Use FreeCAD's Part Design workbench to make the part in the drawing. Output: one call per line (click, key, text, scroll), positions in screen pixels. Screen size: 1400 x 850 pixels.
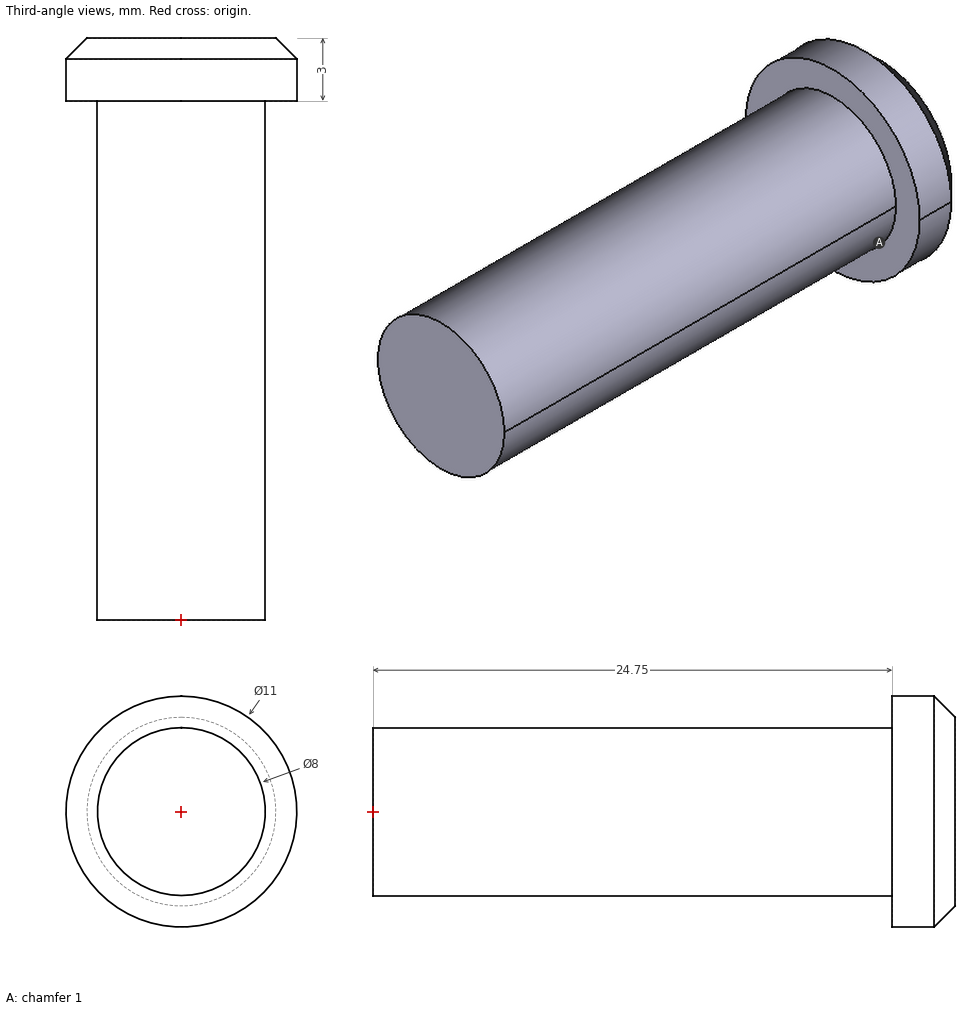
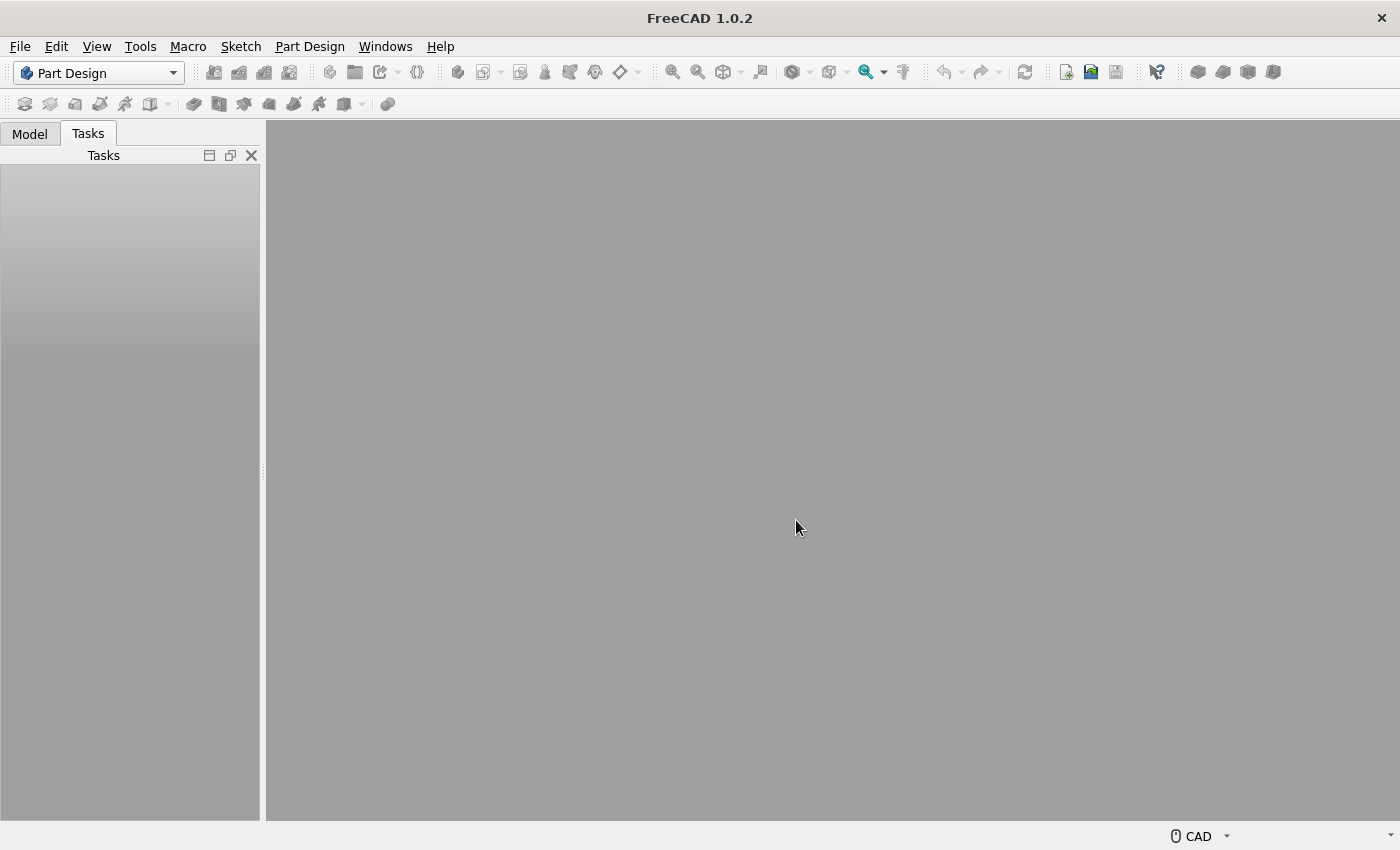
click(1066, 72)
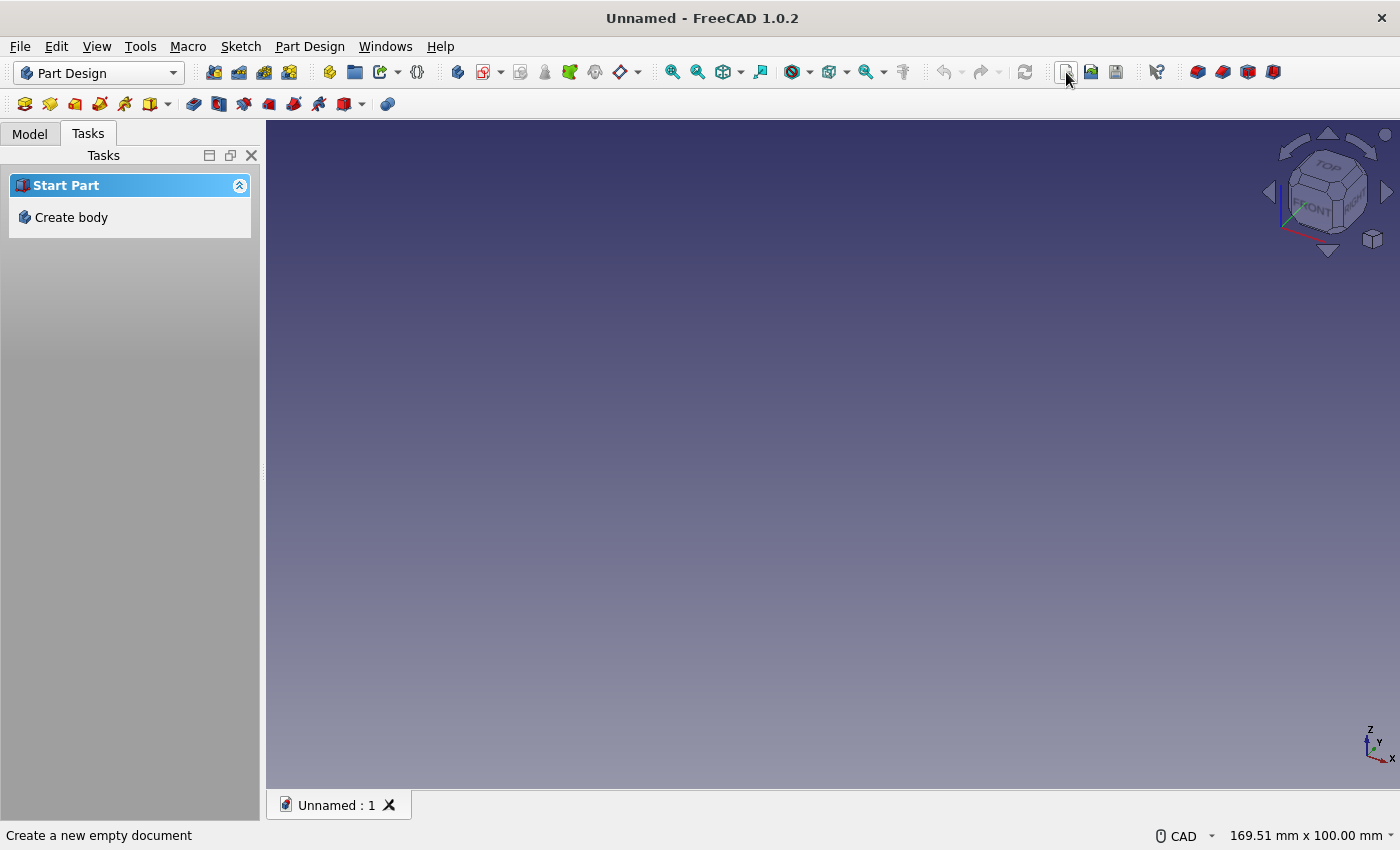
click(482, 72)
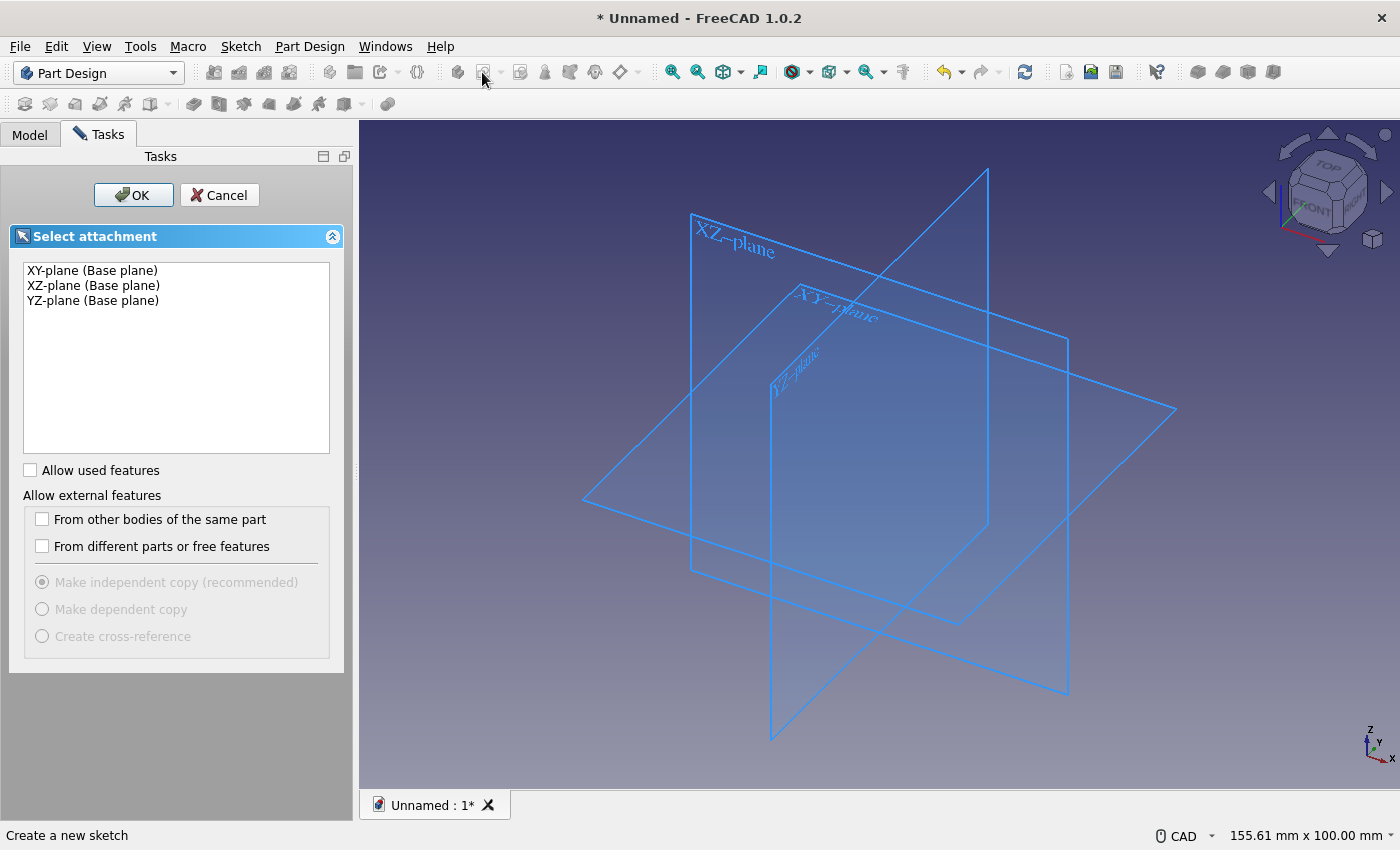
click(84, 286)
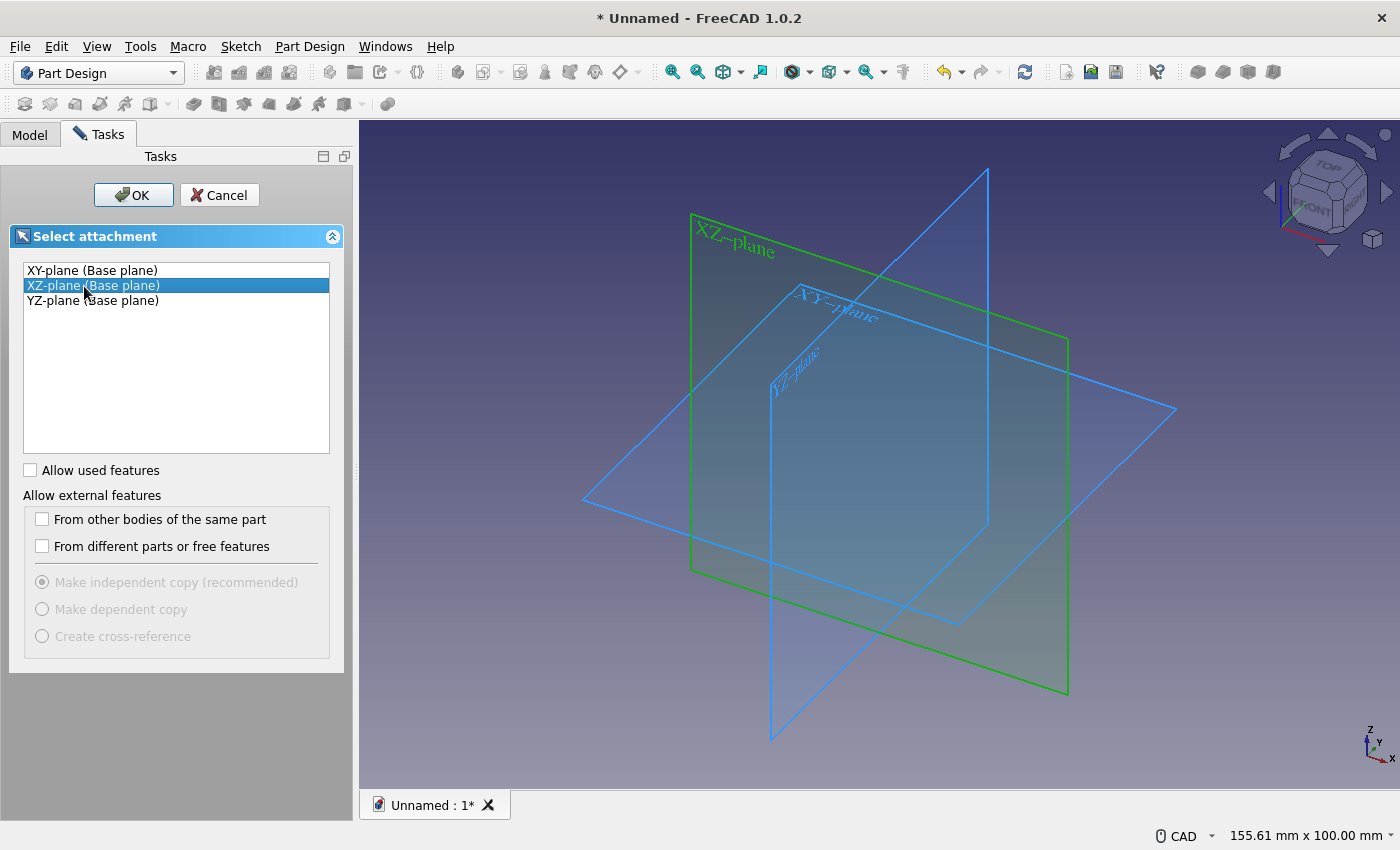
click(134, 195)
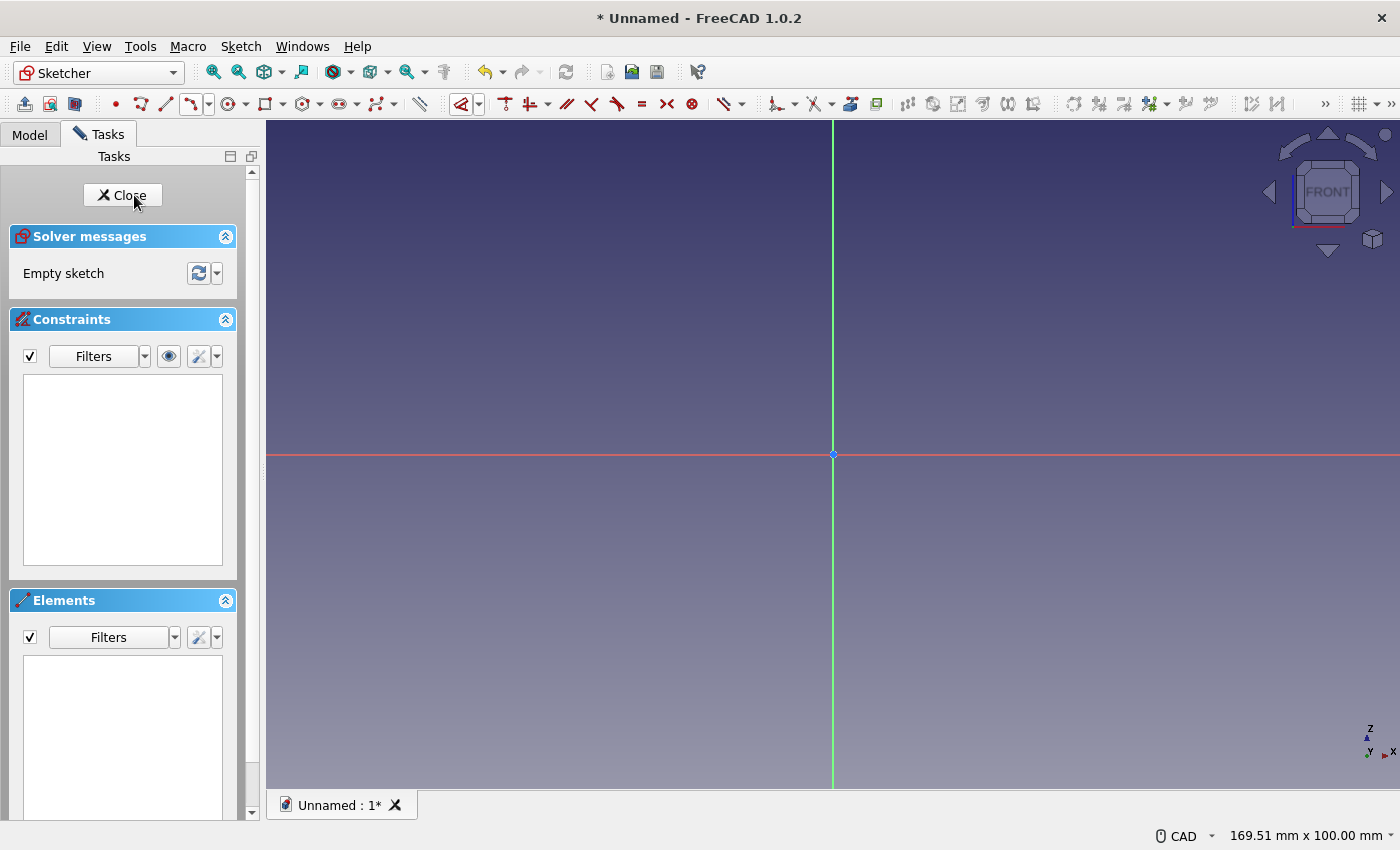
scroll(844, 454, up, 10)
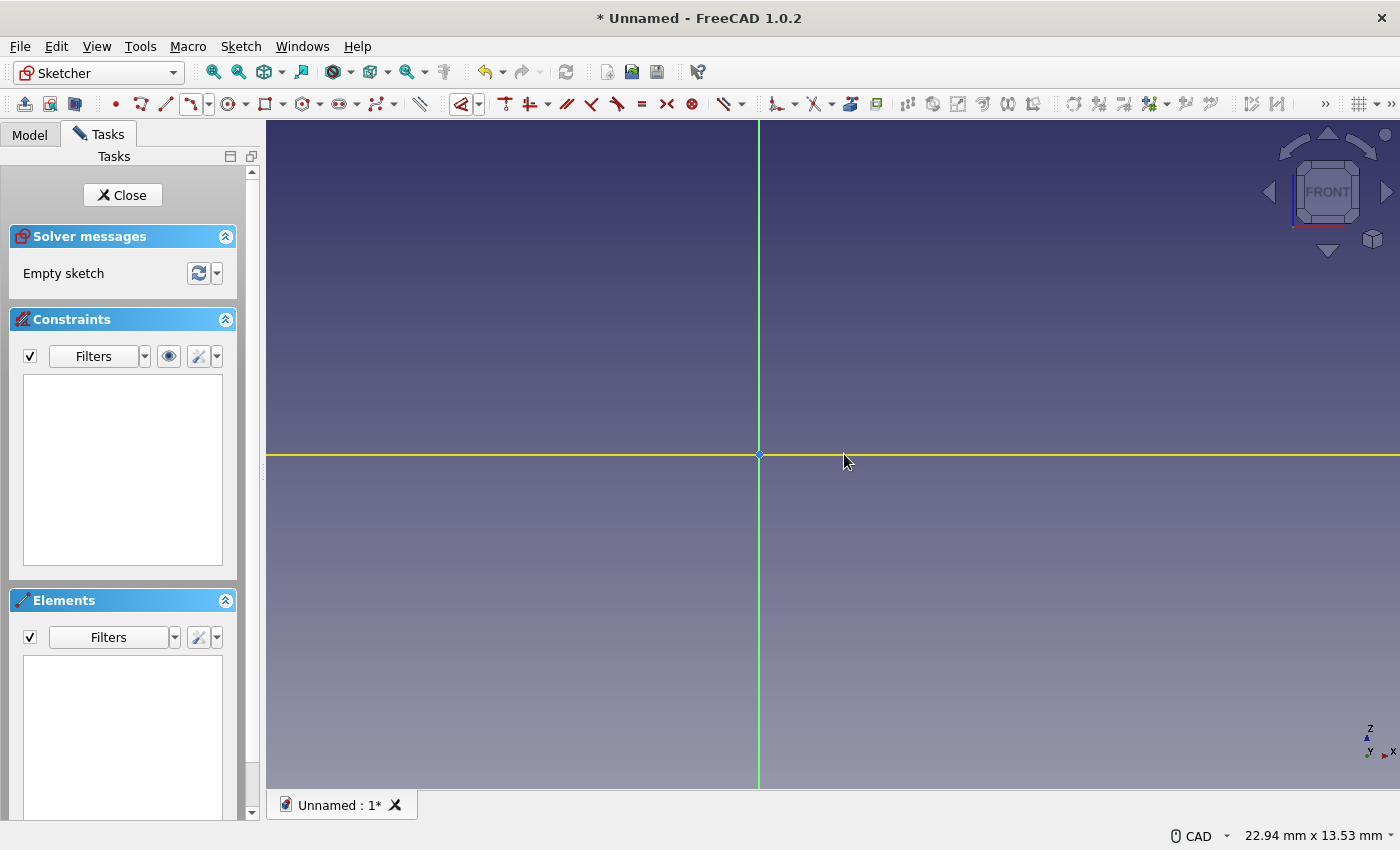
click(228, 104)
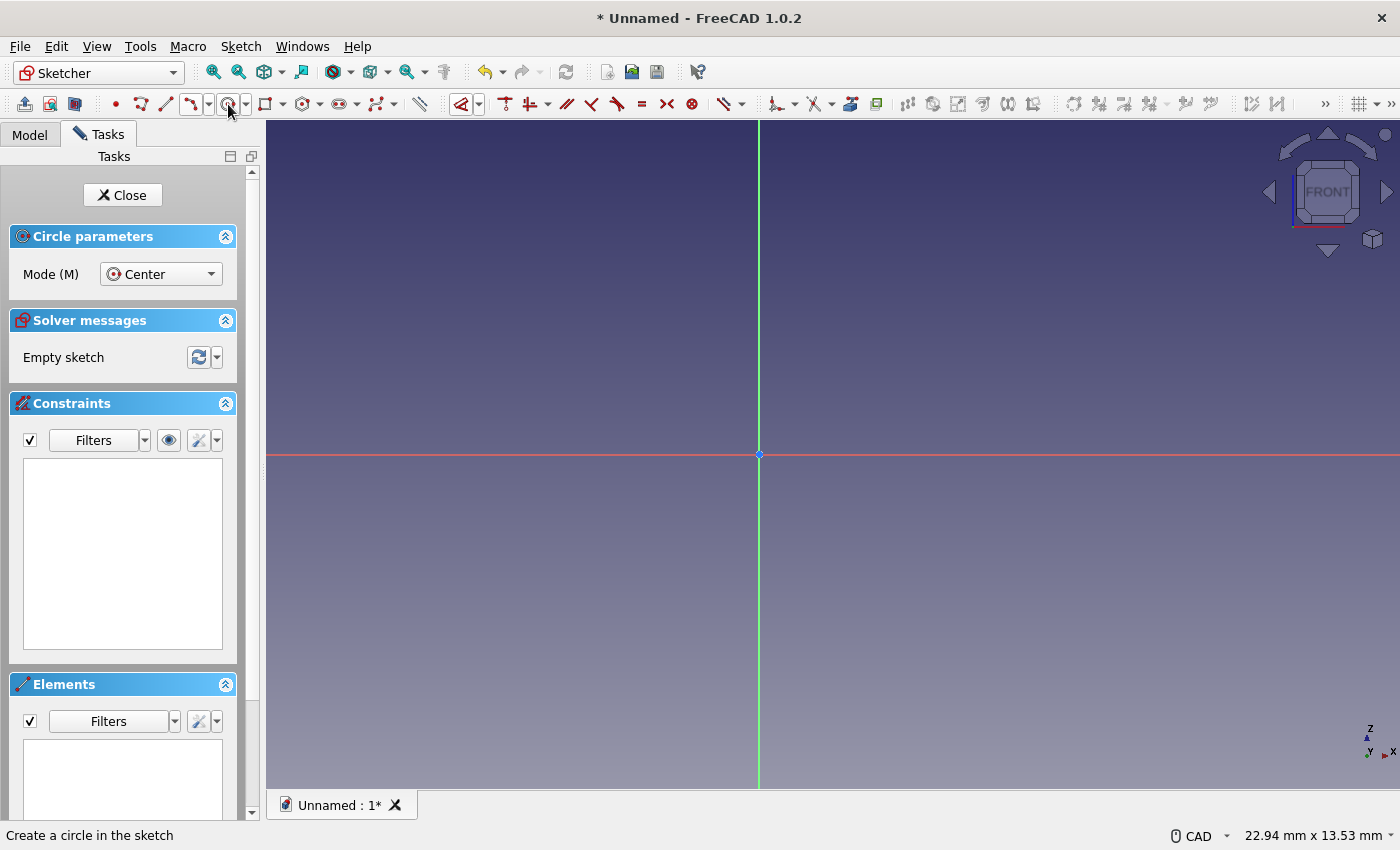
click(759, 454)
click(899, 315)
key(Escape)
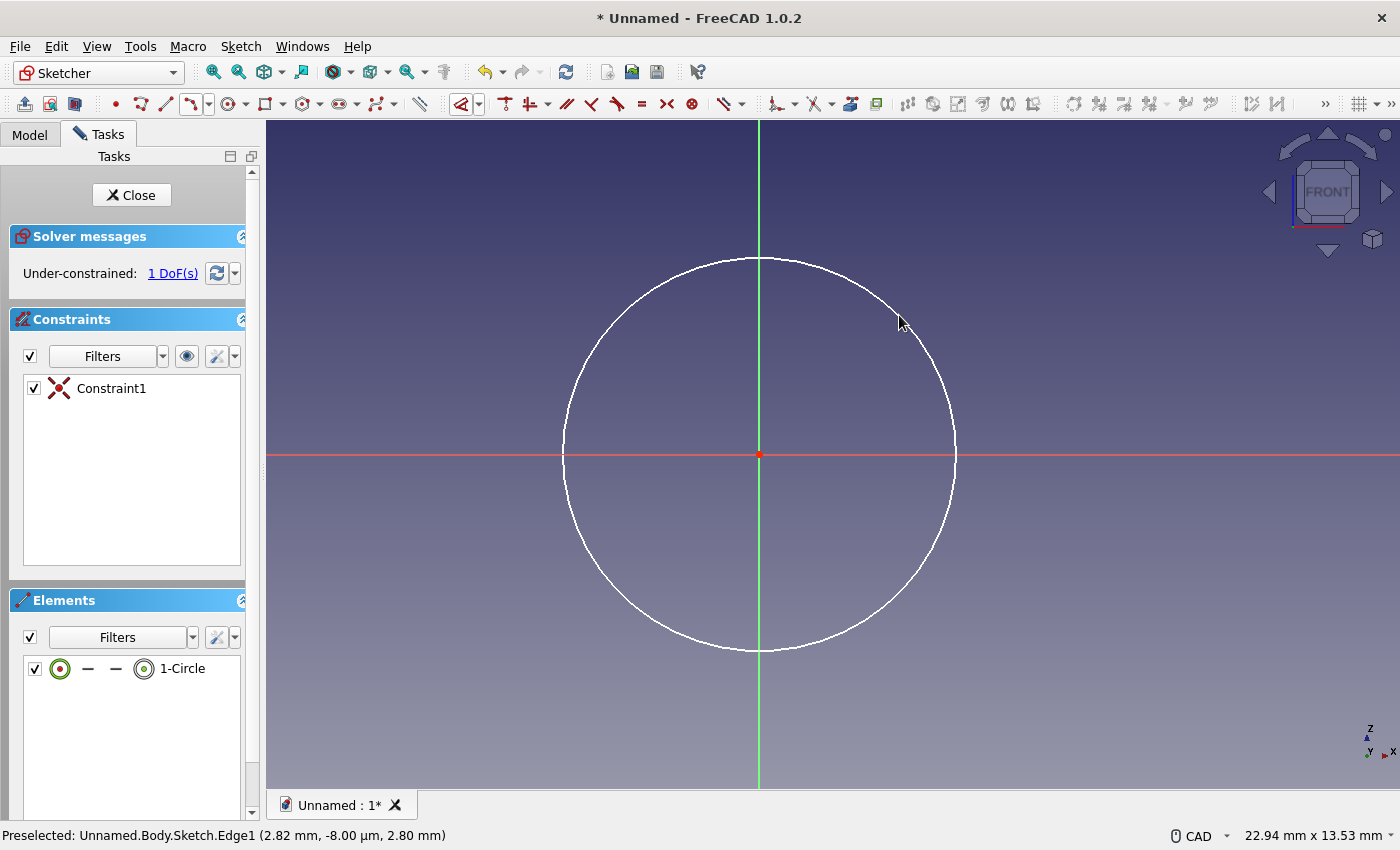
click(460, 104)